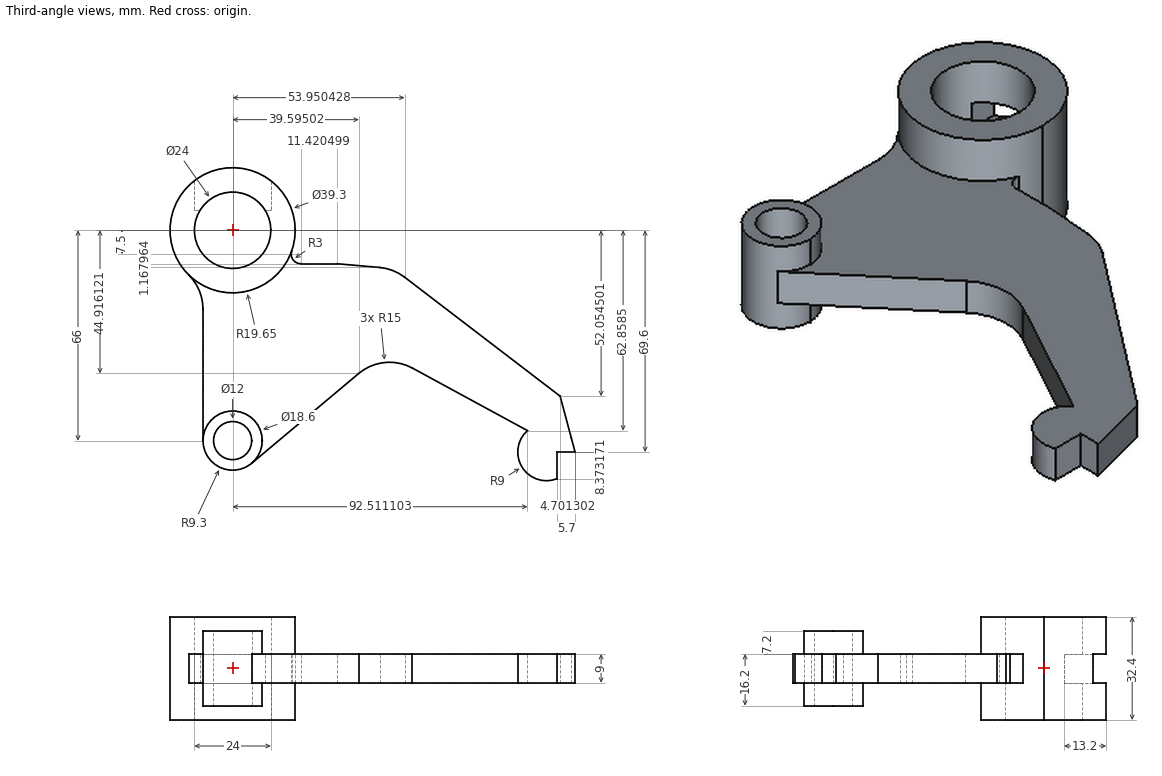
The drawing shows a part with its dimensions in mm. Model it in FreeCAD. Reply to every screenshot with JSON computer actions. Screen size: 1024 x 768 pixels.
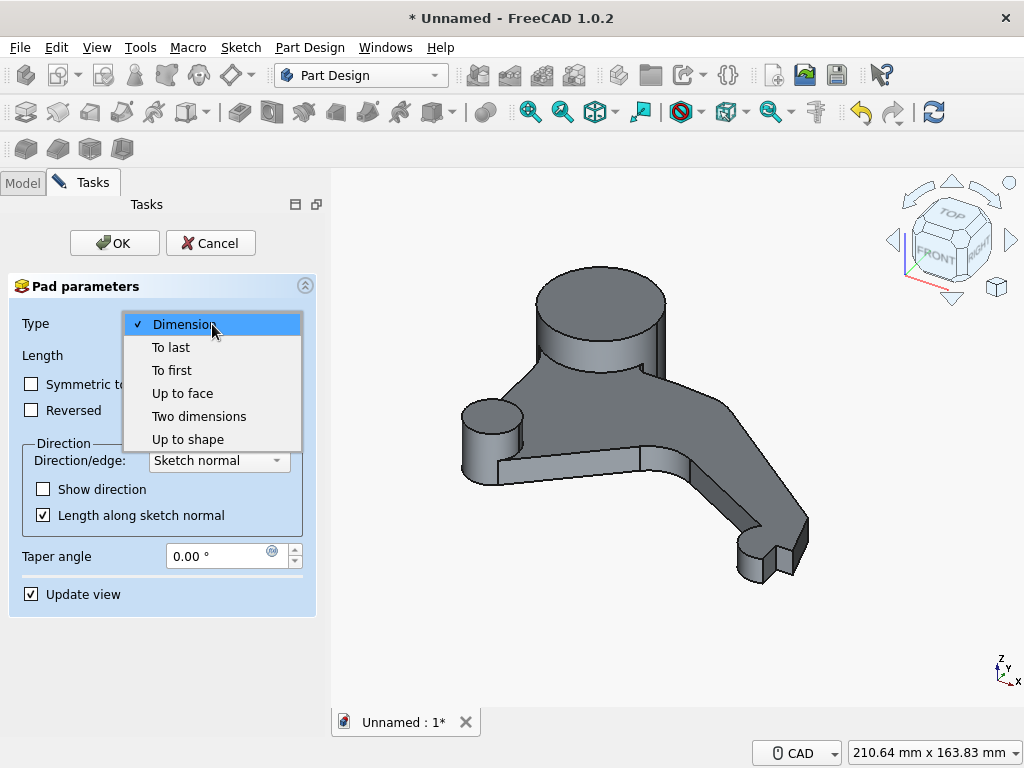
{"action": "left_click", "coordinate": [212, 416]}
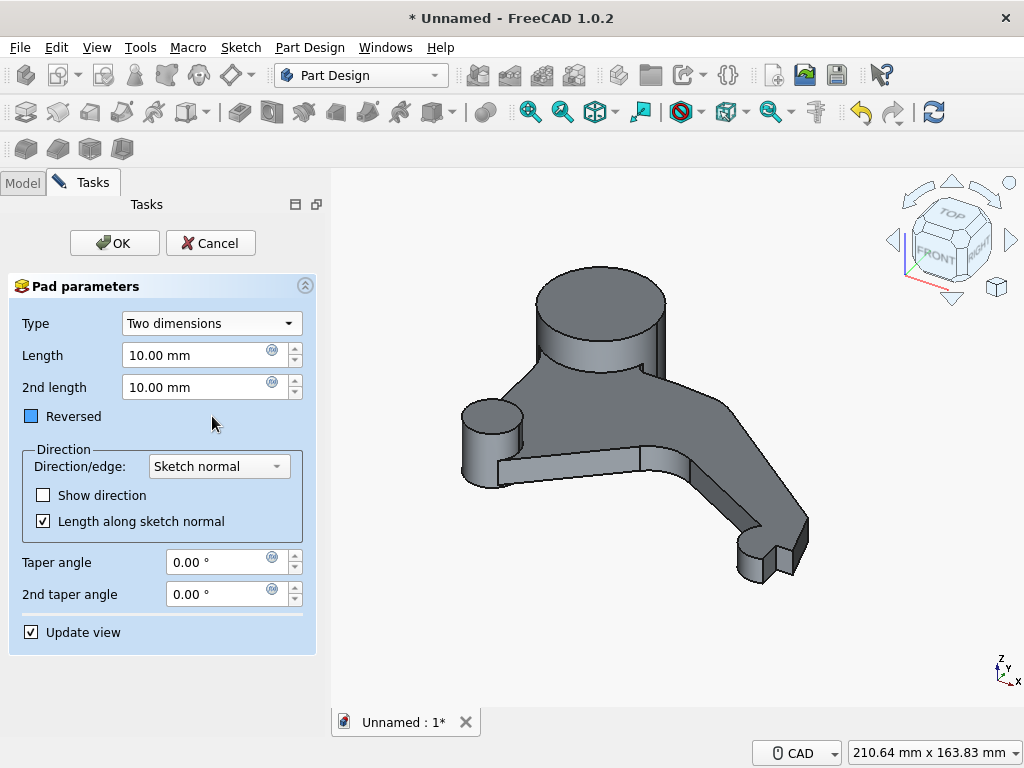
{"action": "triple_click", "coordinate": [204, 355]}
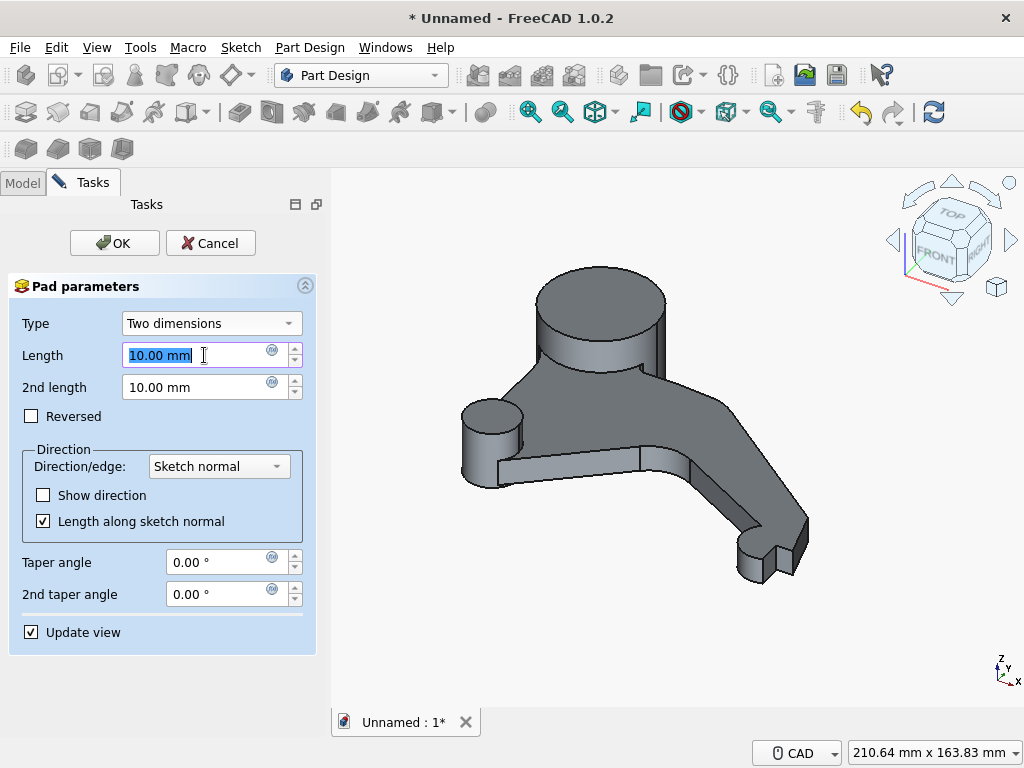
{"action": "type", "text": "7.2"}
{"action": "key", "text": "Tab"}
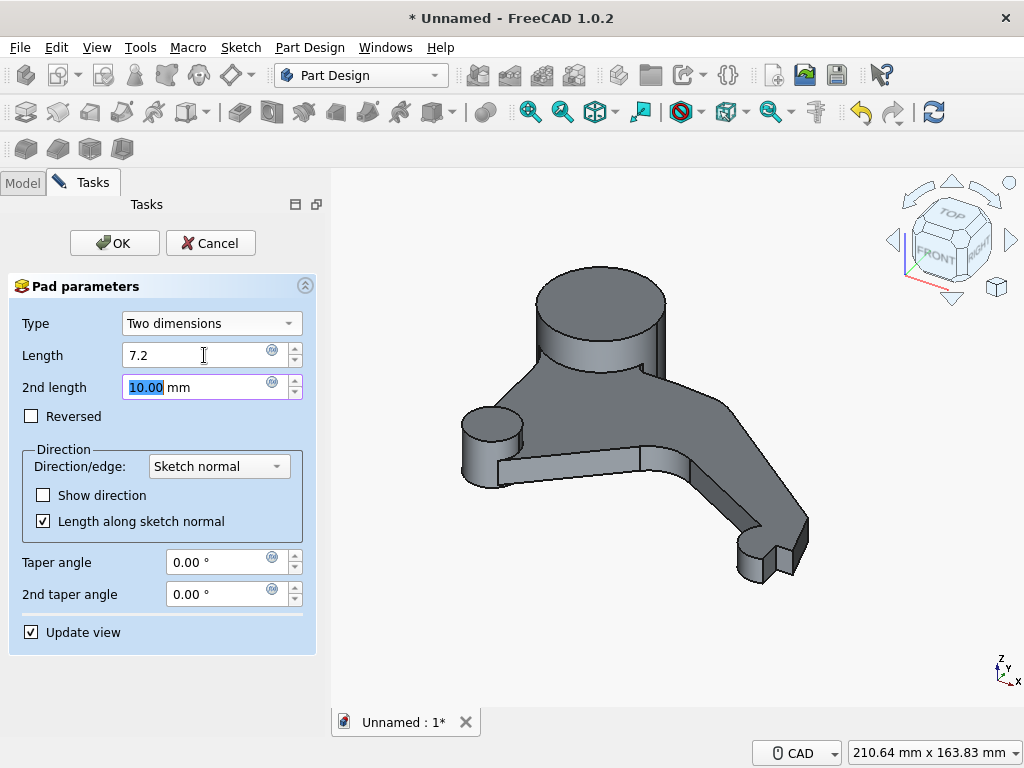
{"action": "type", "text": "16.2"}
{"action": "key", "text": "Tab"}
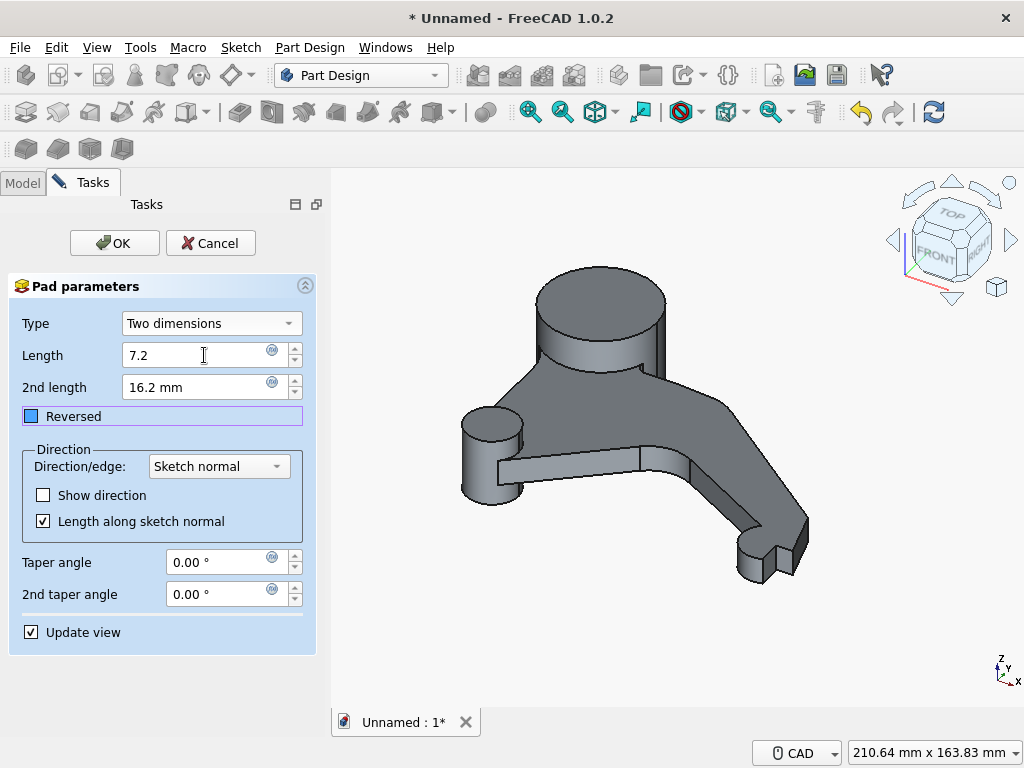
{"action": "left_click", "coordinate": [115, 243]}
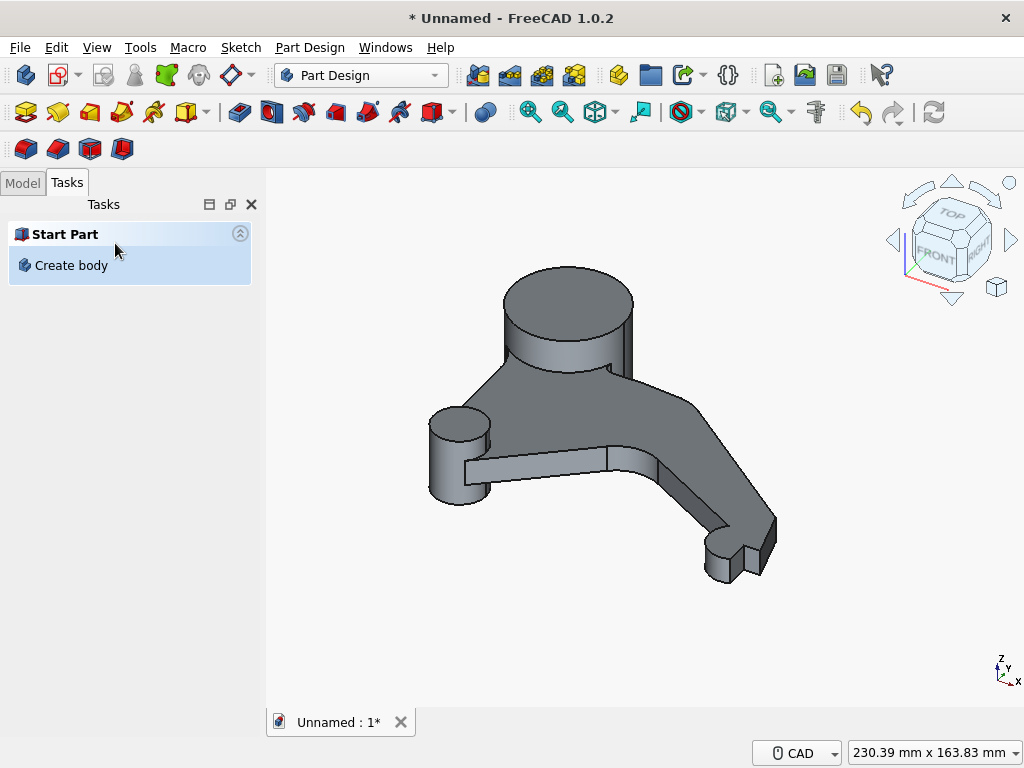
{"action": "left_click", "coordinate": [460, 423]}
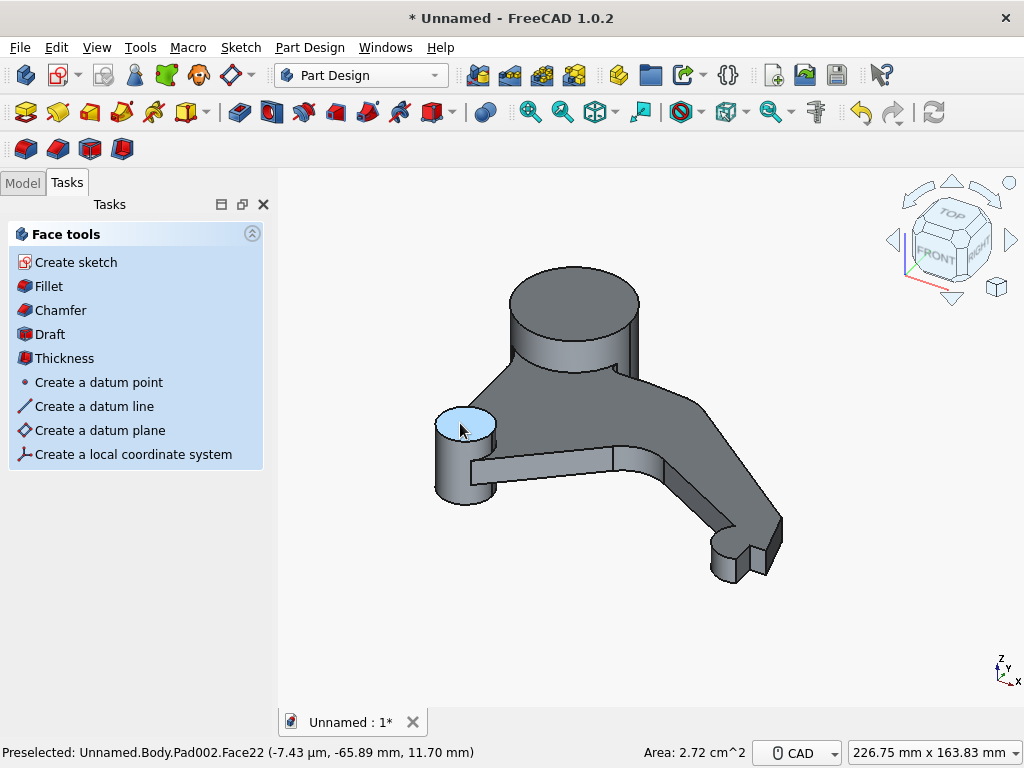
{"action": "left_click", "coordinate": [58, 76]}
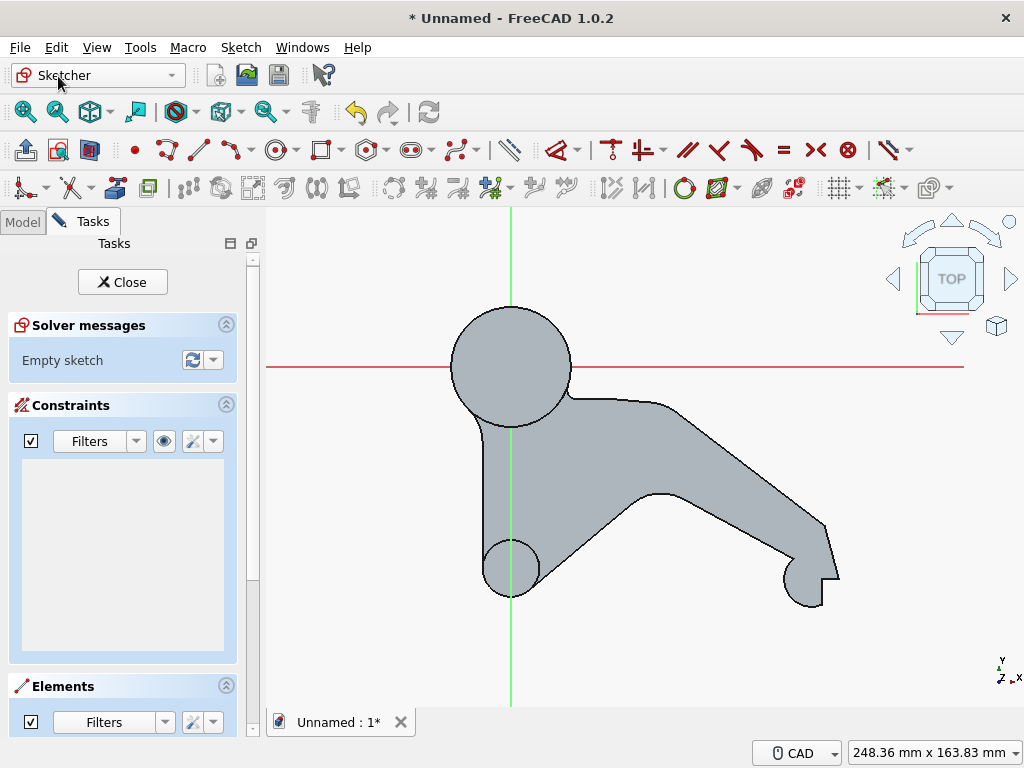
{"action": "key", "text": "q s"}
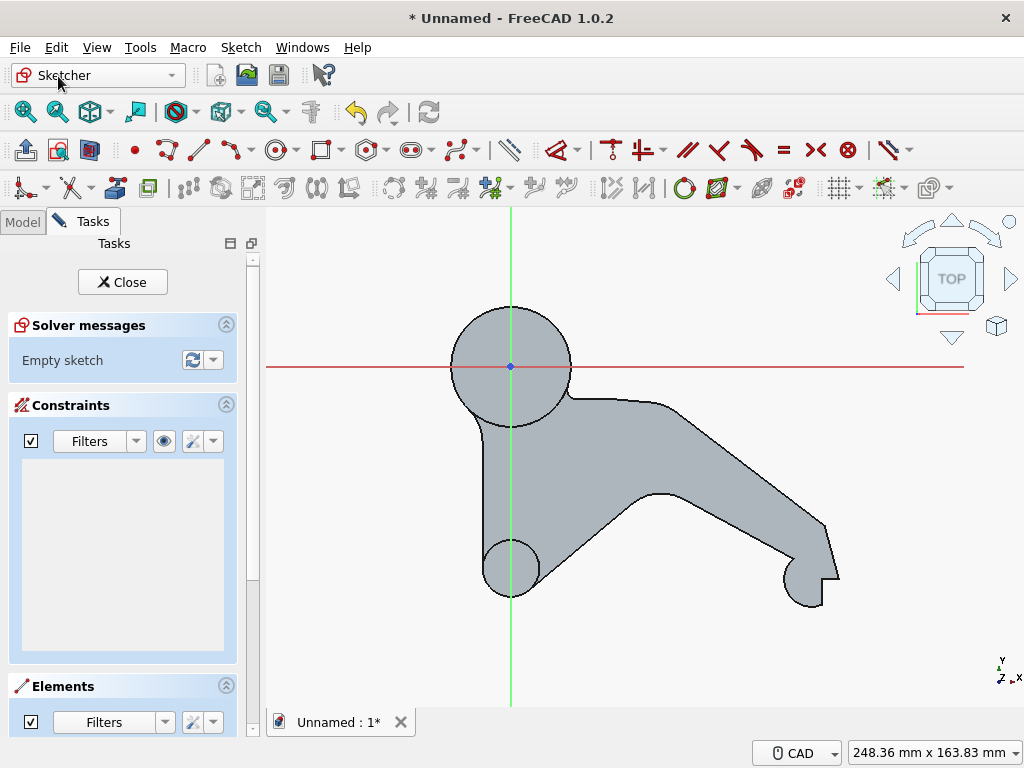
{"action": "scroll", "coordinate": [503, 582], "scroll_direction": "up", "scroll_amount": 11}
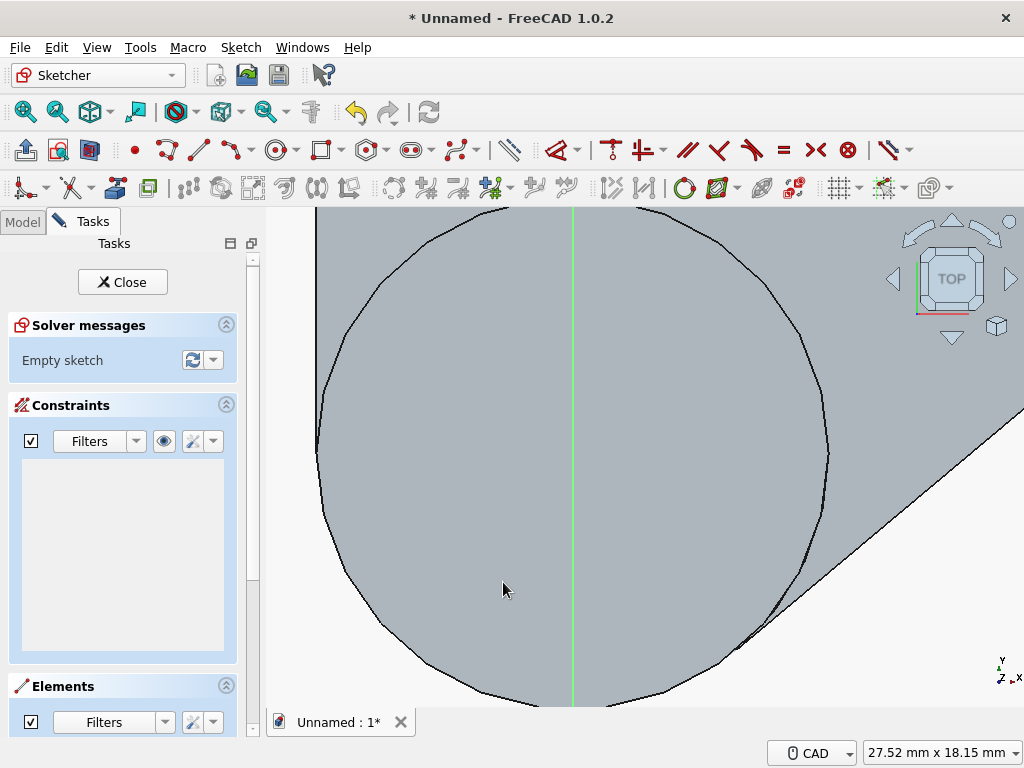
{"action": "key", "text": "g c"}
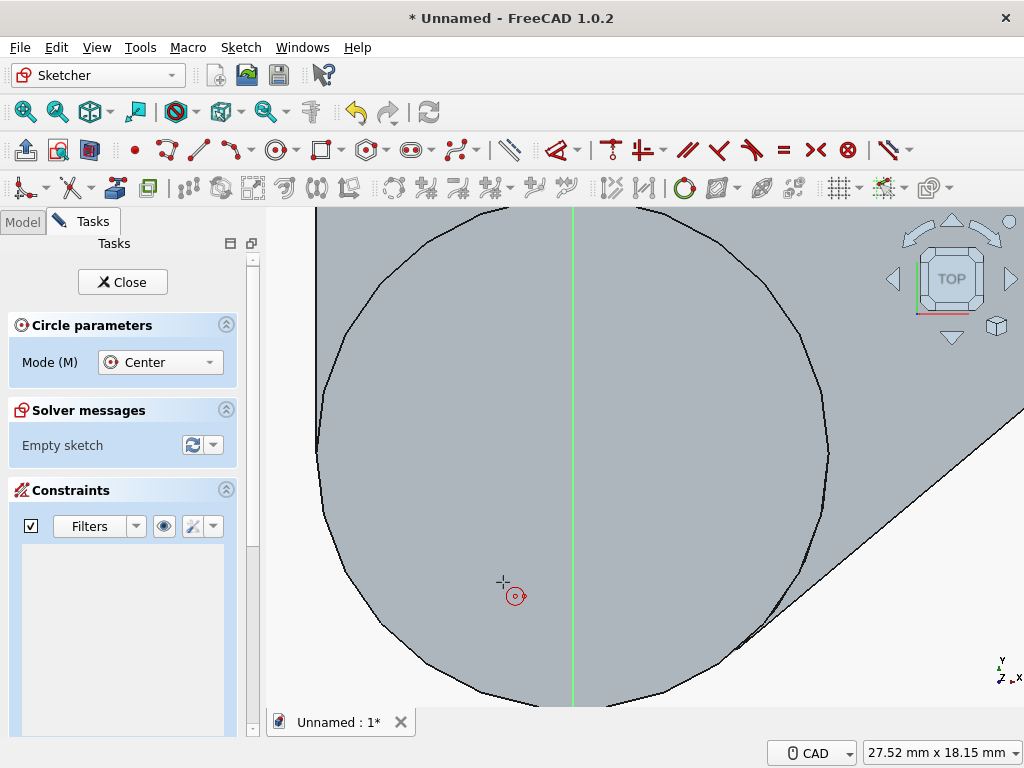
{"action": "left_click", "coordinate": [573, 453]}
{"action": "mouse_move", "coordinate": [689, 336]}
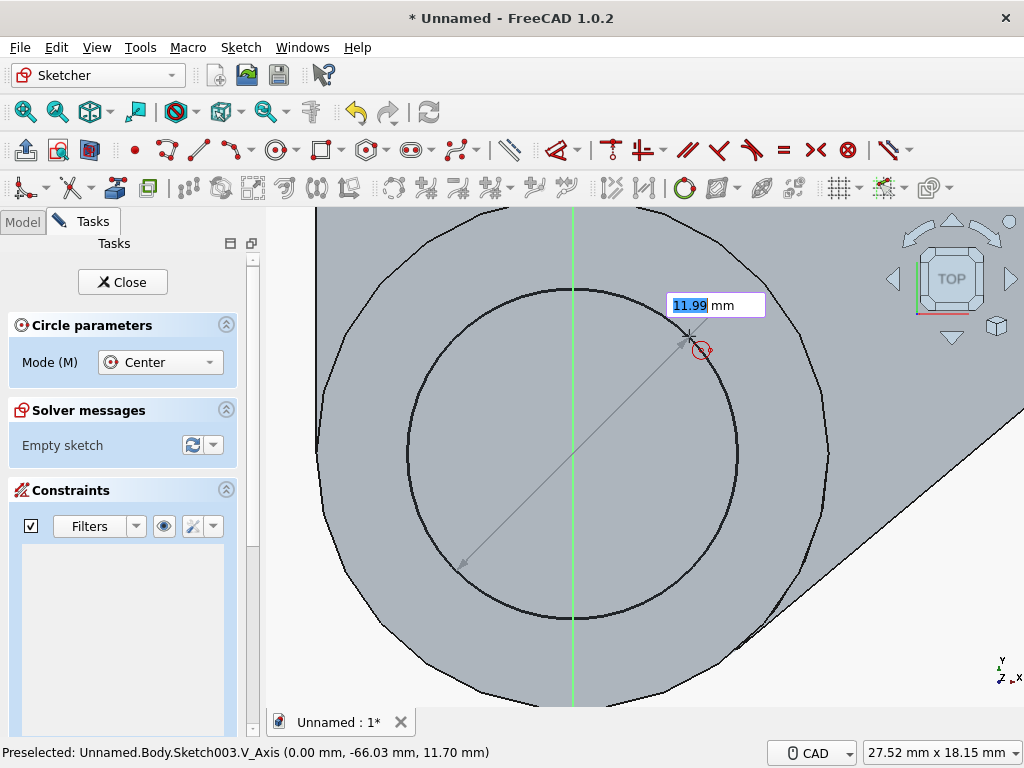
{"action": "type", "text": "12"}
{"action": "key", "text": "Return"}
{"action": "key", "text": "Escape"}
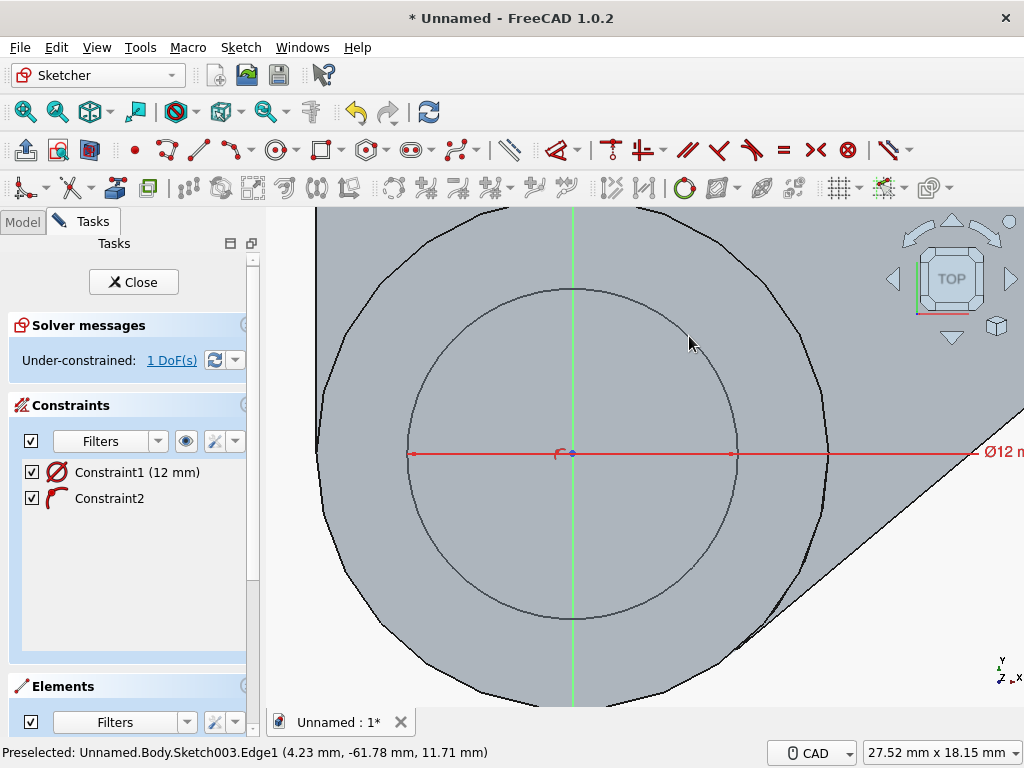
{"action": "key", "text": "d"}